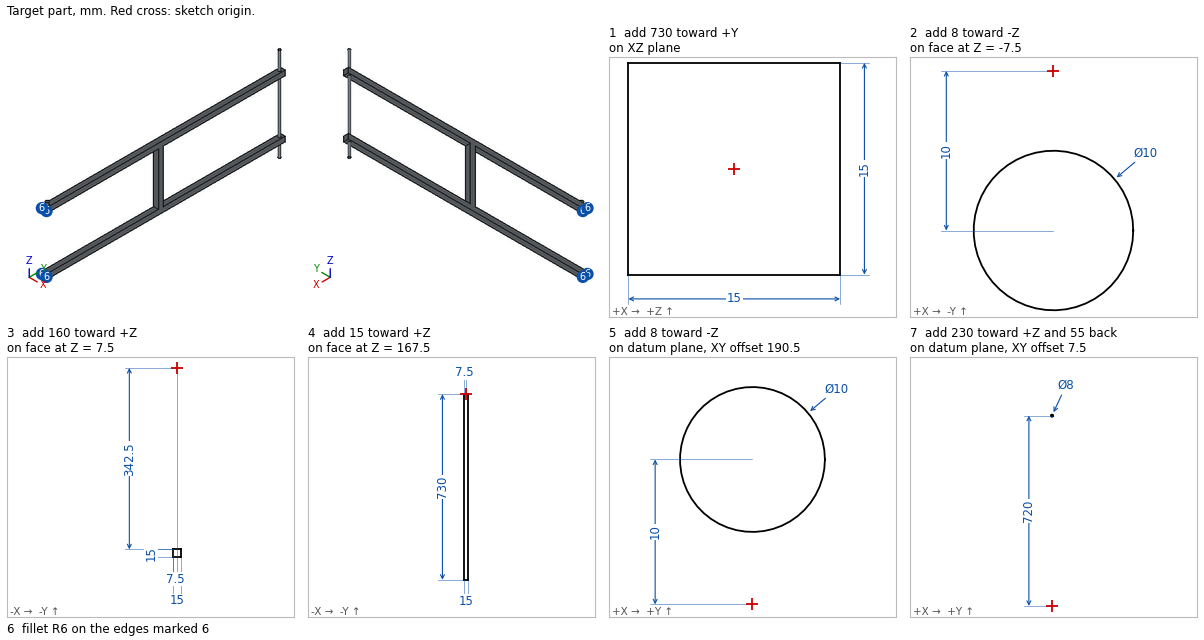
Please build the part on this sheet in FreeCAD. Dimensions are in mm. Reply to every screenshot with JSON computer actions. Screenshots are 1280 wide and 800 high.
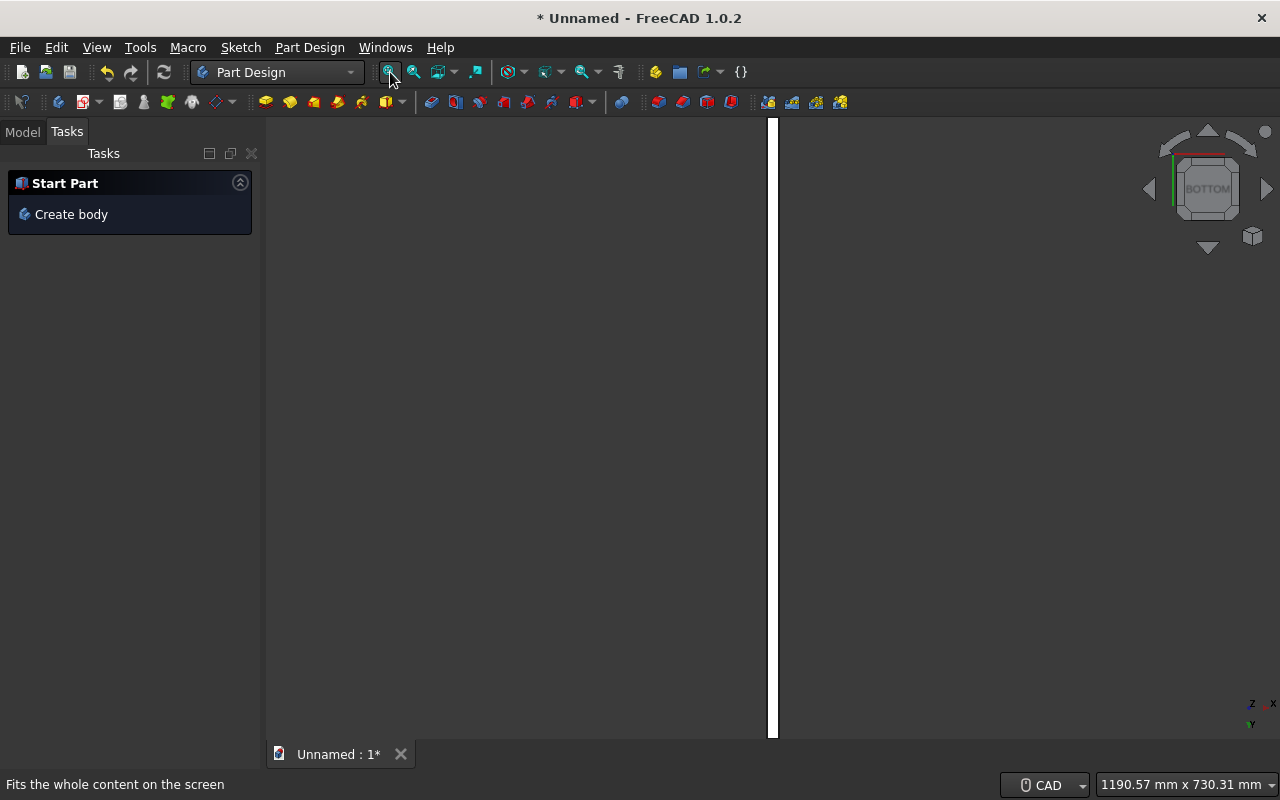
{"action": "left_click", "coordinate": [390, 72]}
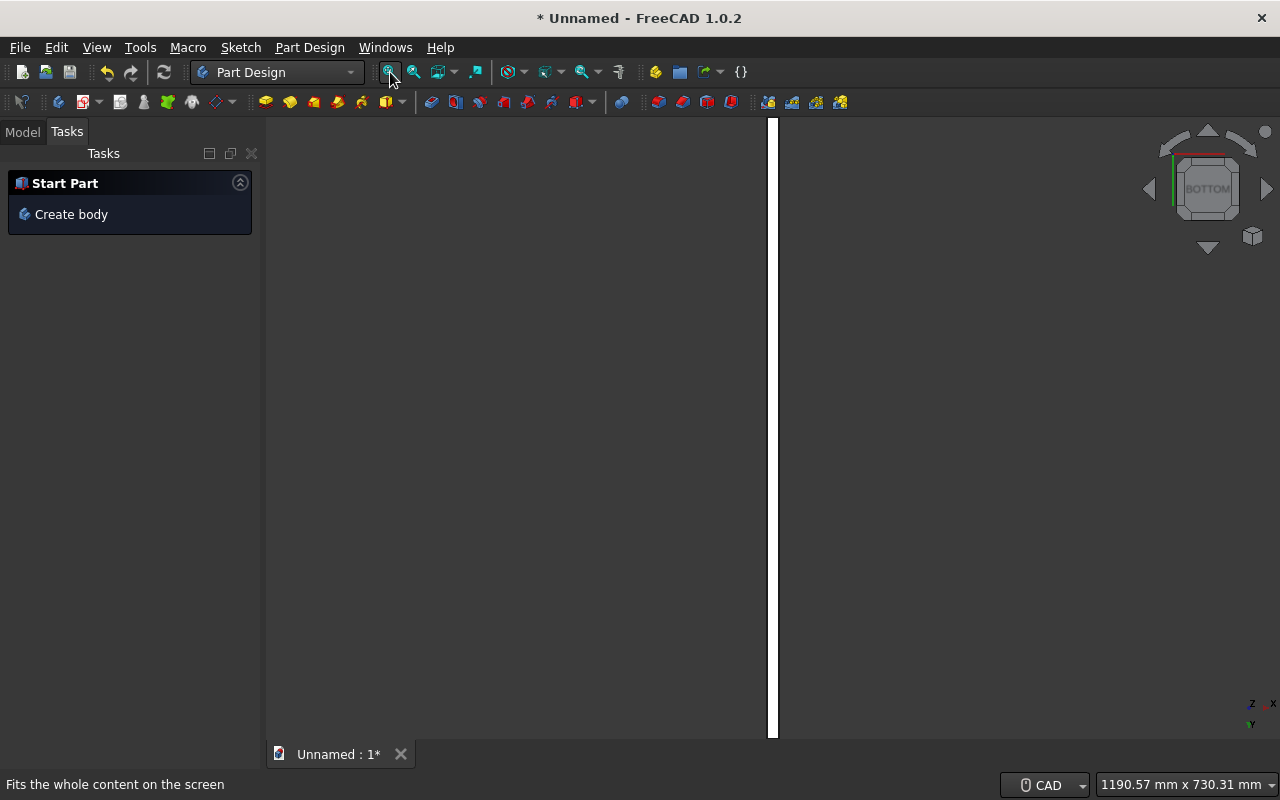
{"action": "scroll", "coordinate": [773, 693], "scroll_direction": "up", "scroll_amount": 4}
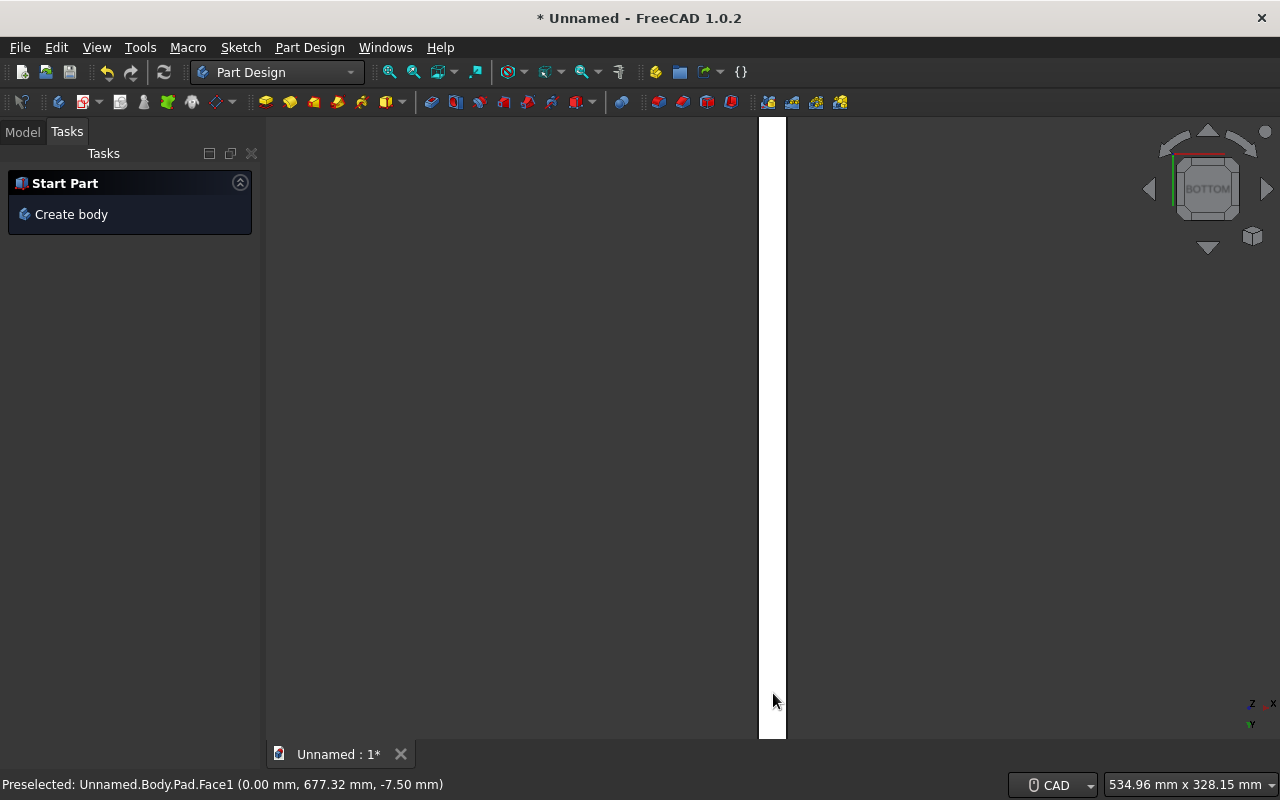
{"action": "left_click", "coordinate": [772, 694]}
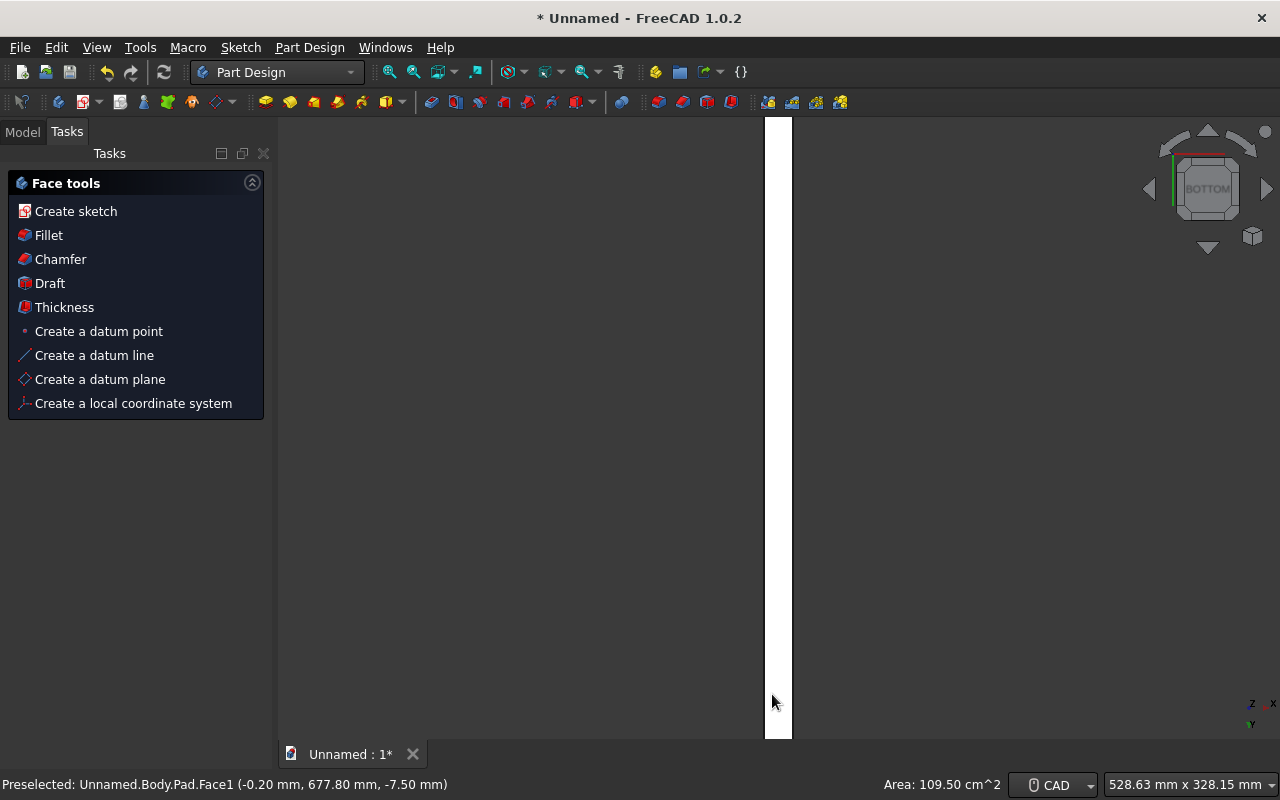
{"action": "left_click", "coordinate": [84, 102]}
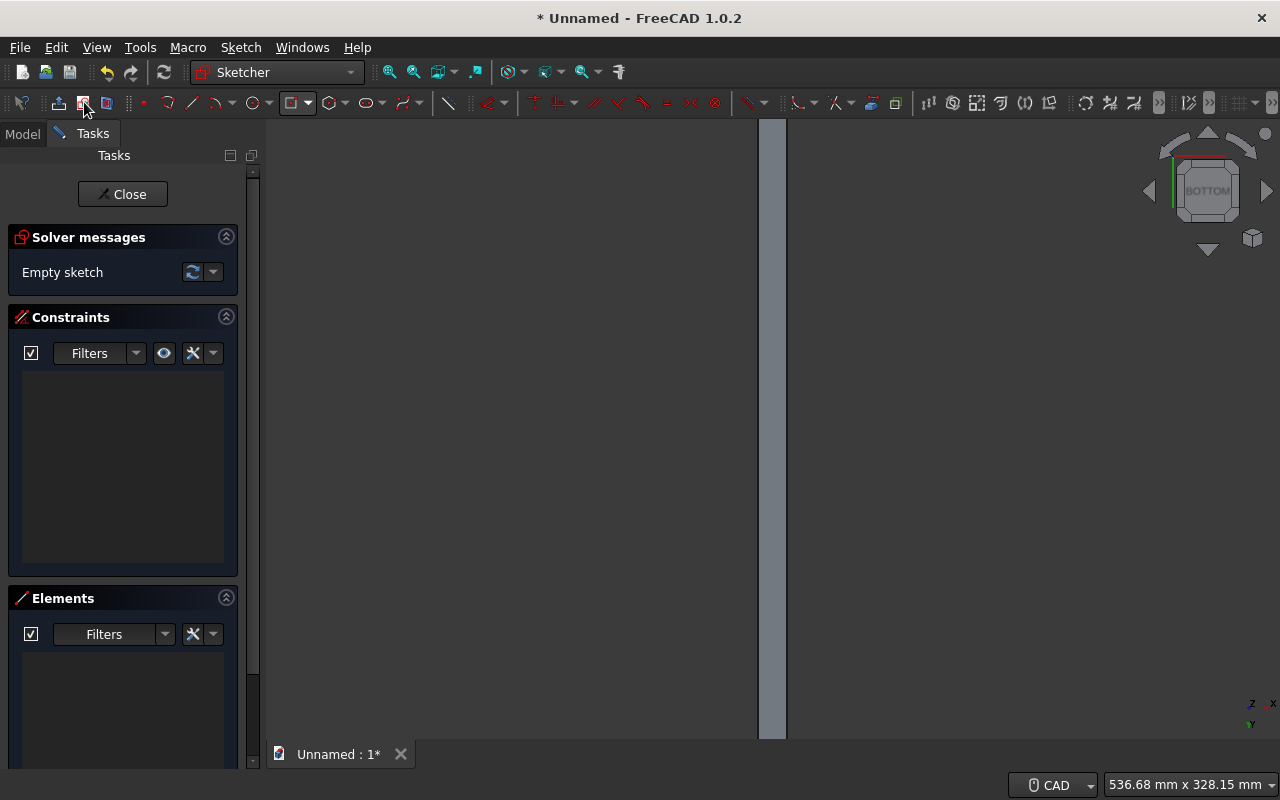
{"action": "scroll", "coordinate": [704, 429], "scroll_direction": "down", "scroll_amount": 5}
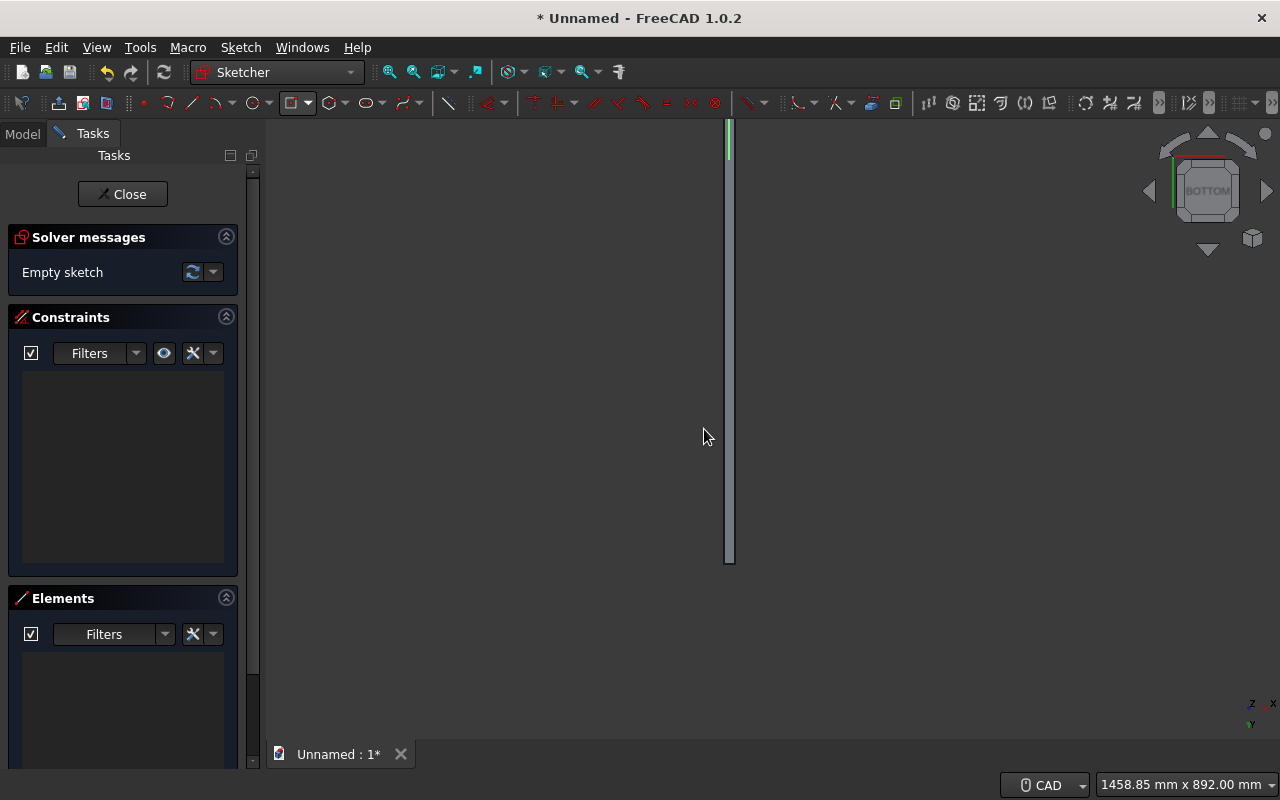
{"action": "scroll", "coordinate": [704, 429], "scroll_direction": "down", "scroll_amount": 5}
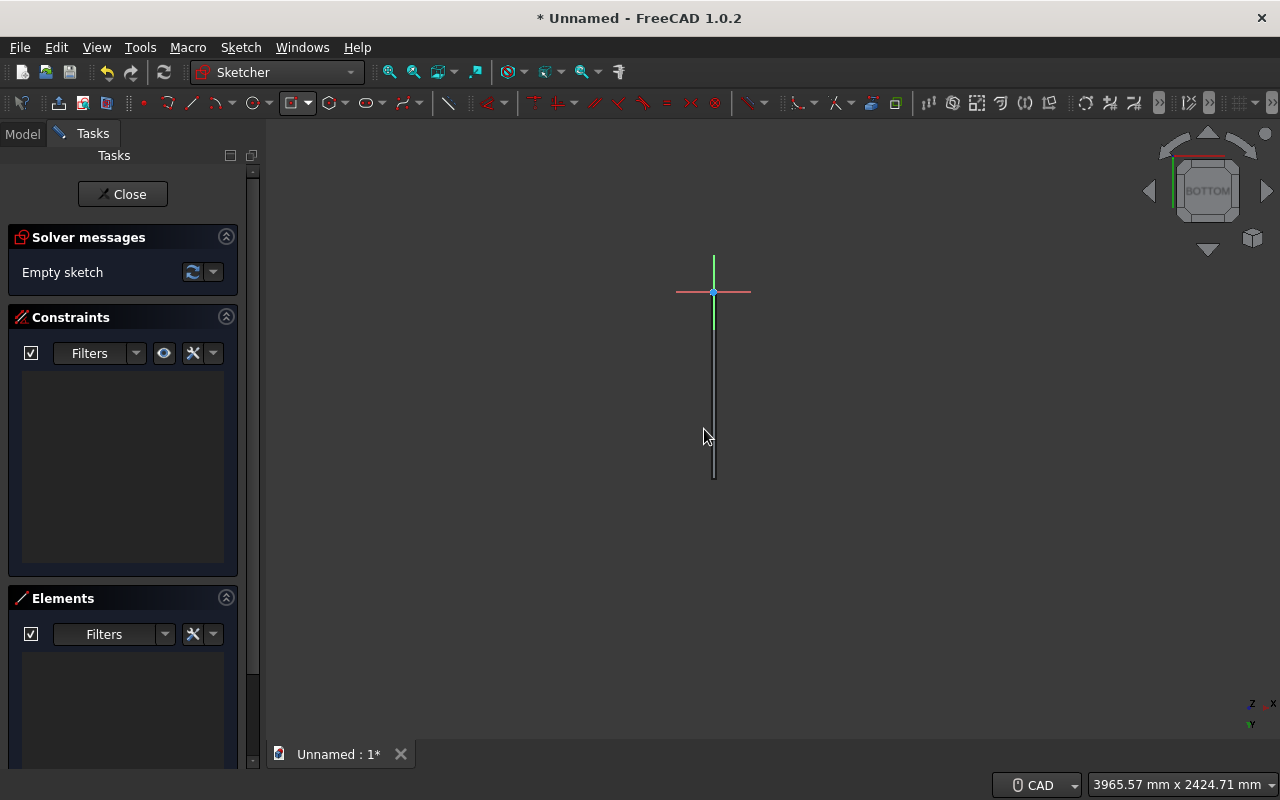
{"action": "scroll", "coordinate": [714, 287], "scroll_direction": "up", "scroll_amount": 15}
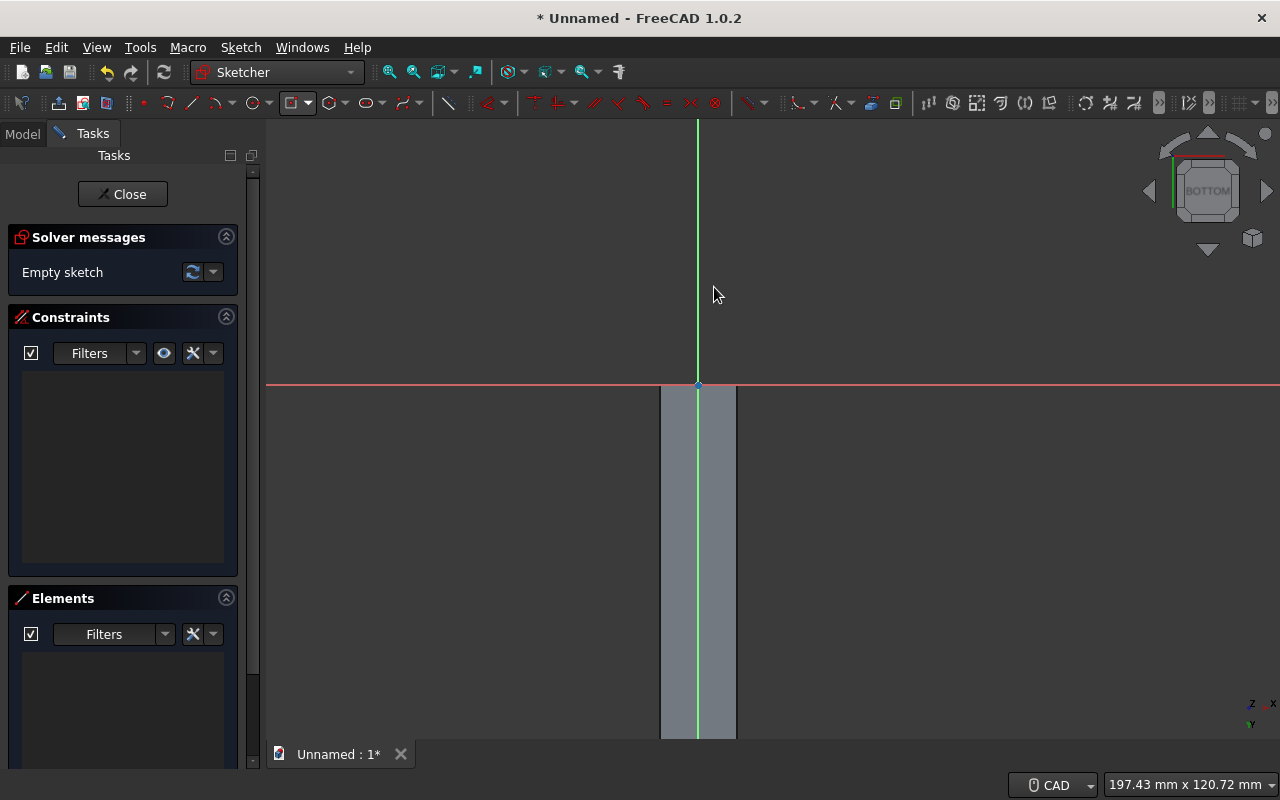
{"action": "scroll", "coordinate": [696, 422], "scroll_direction": "up", "scroll_amount": 8}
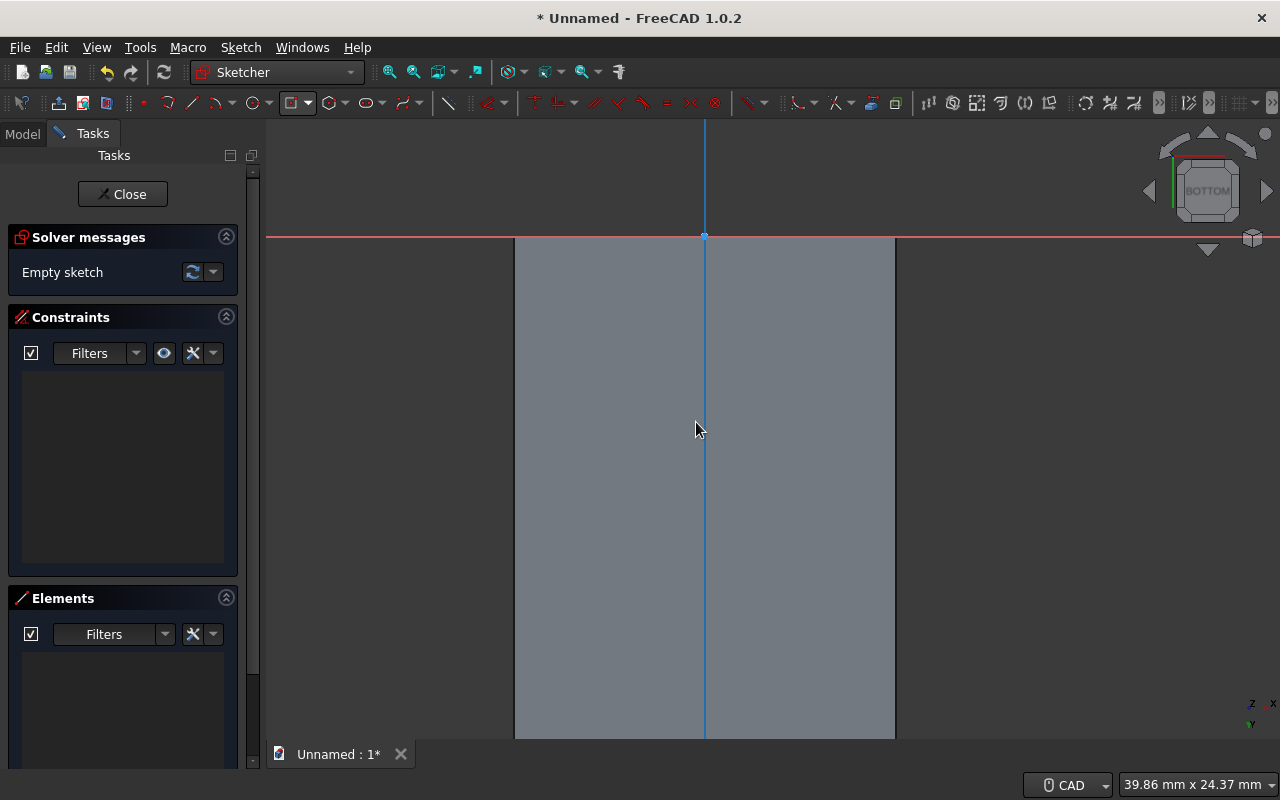
{"action": "left_click", "coordinate": [254, 104]}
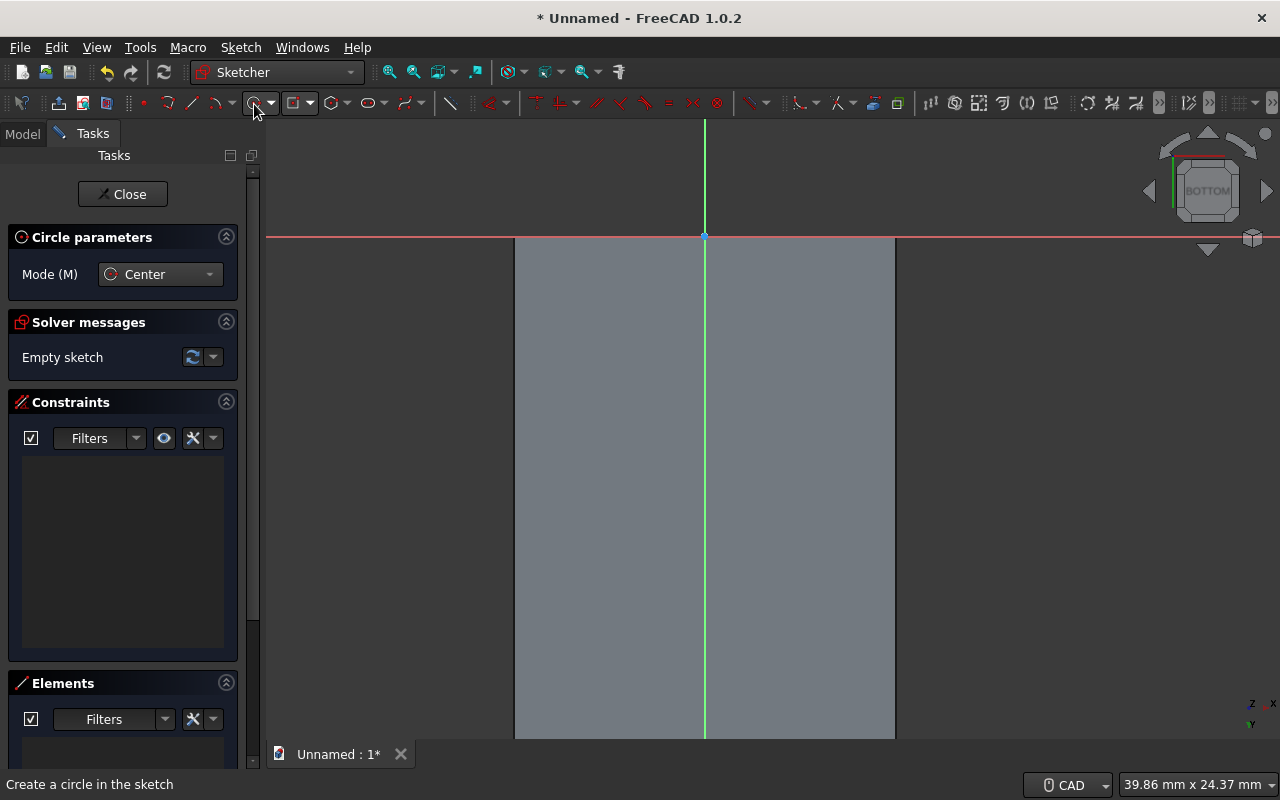
{"action": "left_click", "coordinate": [705, 491]}
{"action": "left_click", "coordinate": [795, 401]}
{"action": "key", "text": "Escape"}